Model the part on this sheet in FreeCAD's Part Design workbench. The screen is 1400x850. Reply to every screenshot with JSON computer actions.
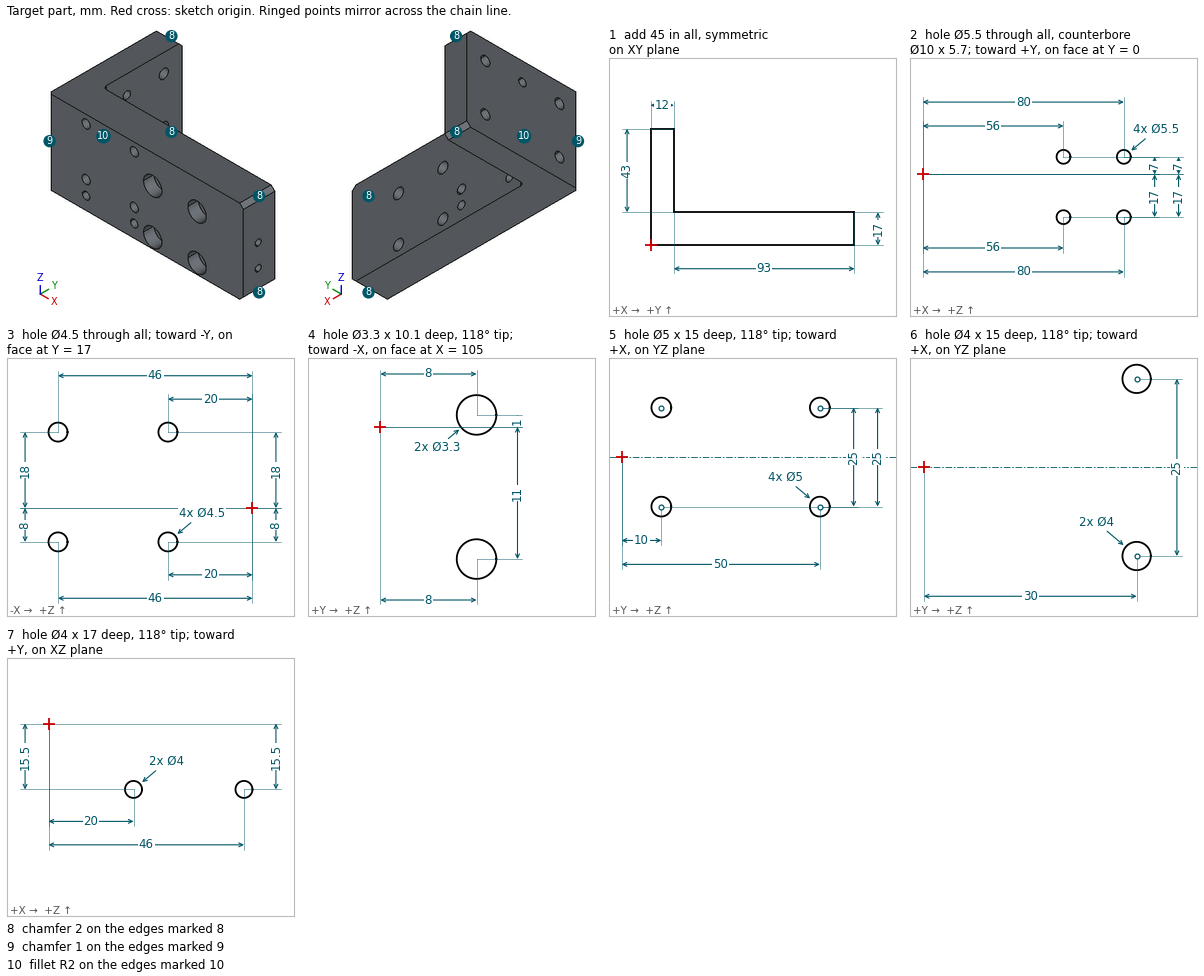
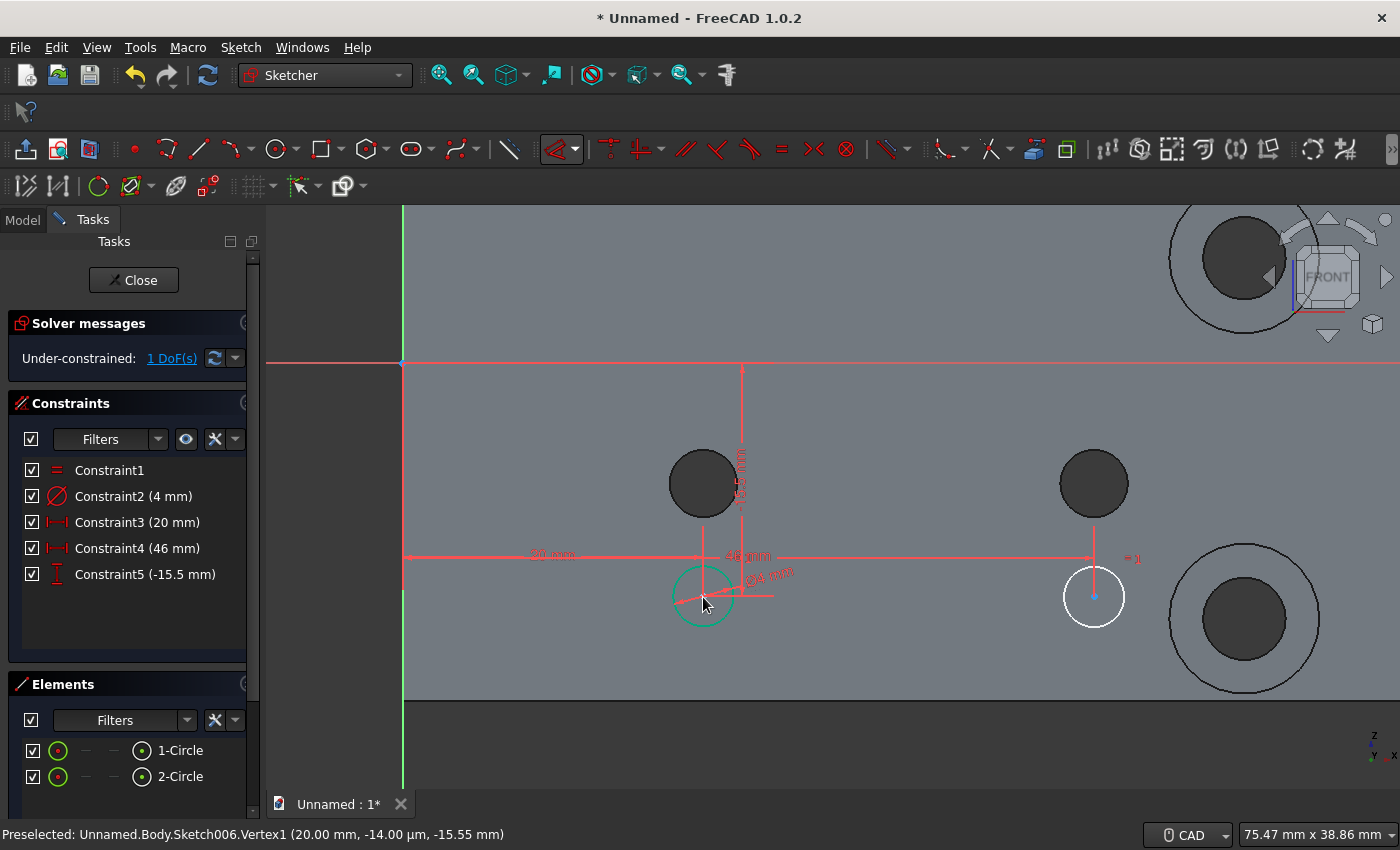
{"action": "left_click", "coordinate": [1094, 597]}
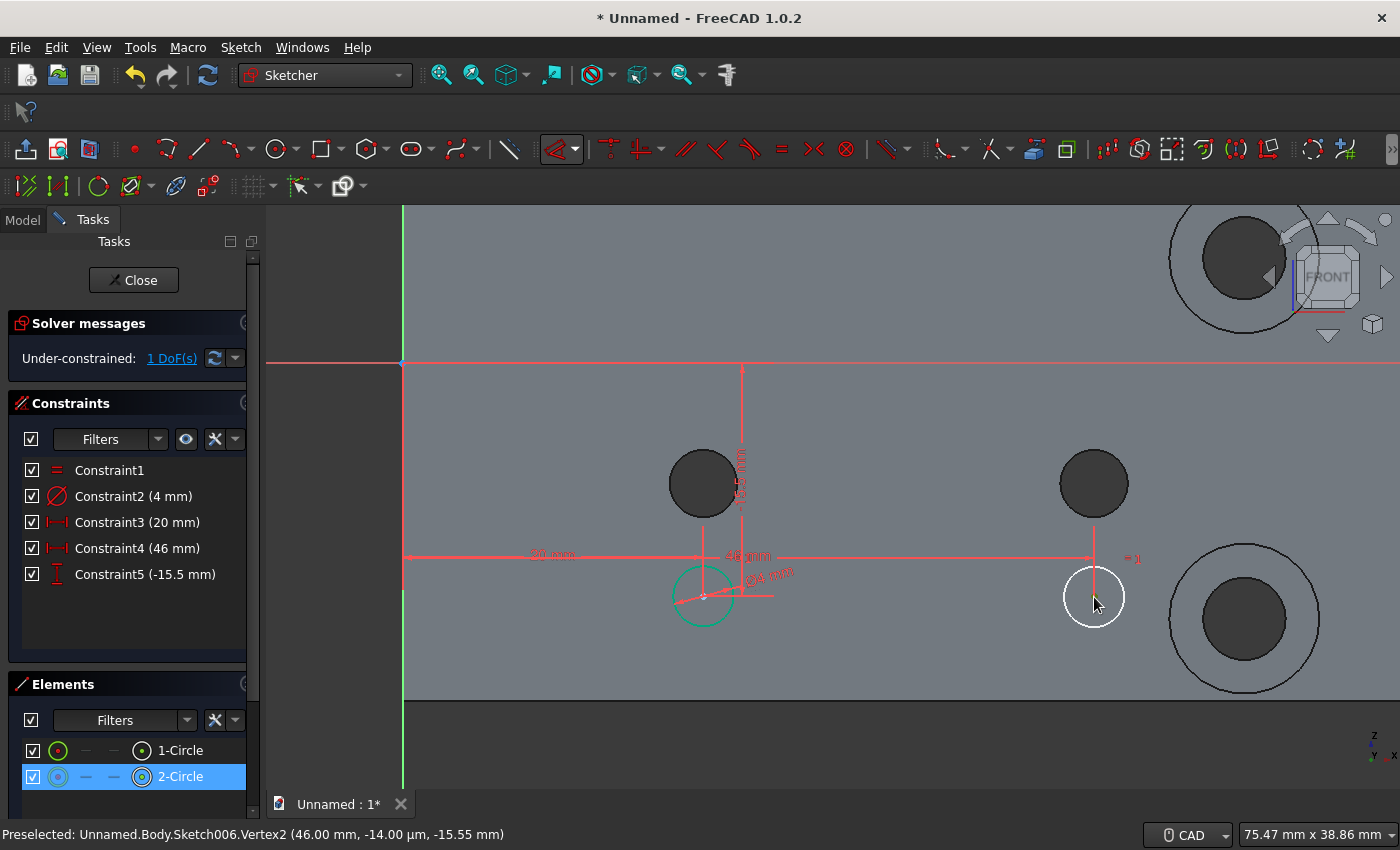
{"action": "key", "text": "i"}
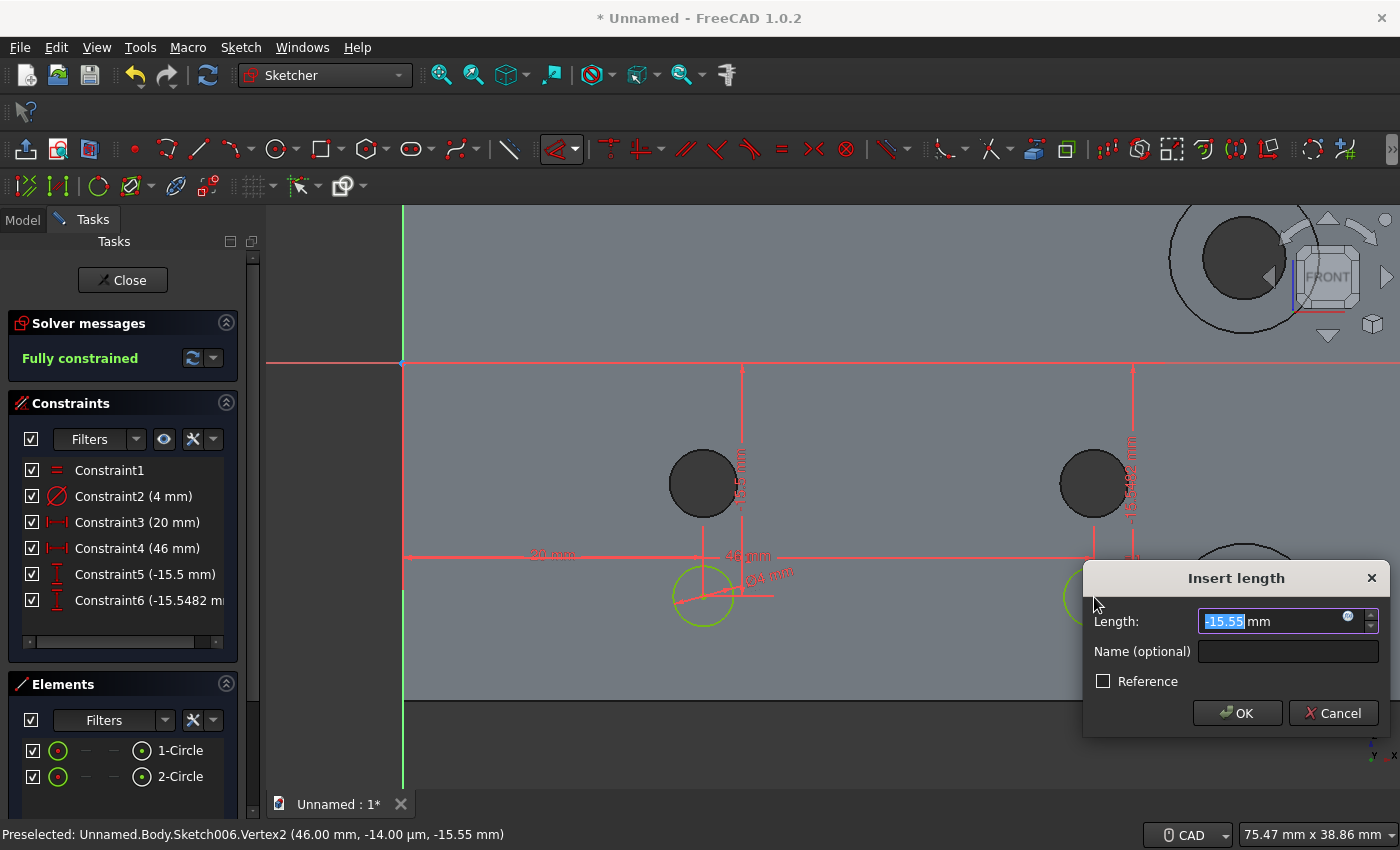
{"action": "type", "text": "-15.5"}
{"action": "key", "text": "Return"}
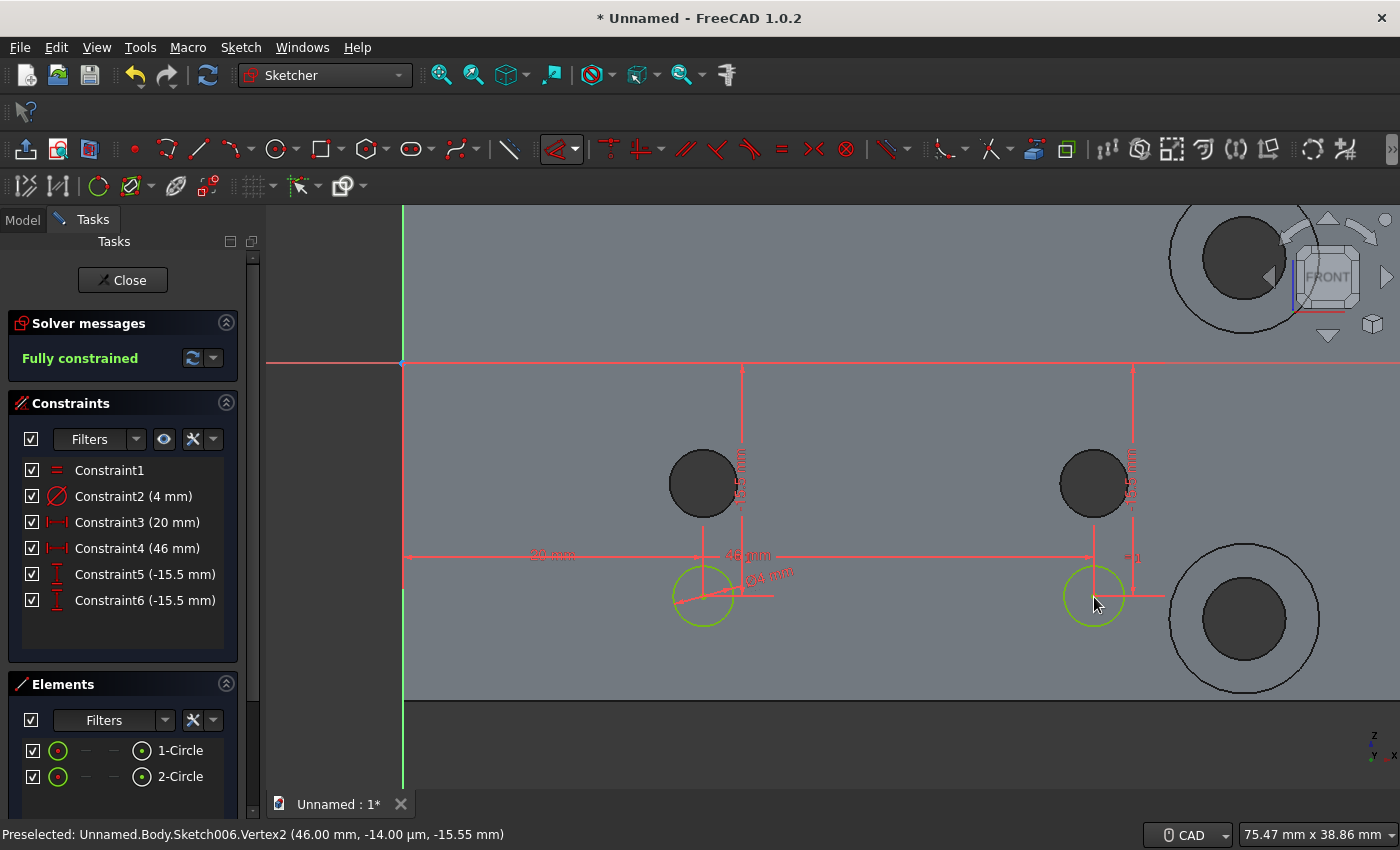
{"action": "left_click", "coordinate": [123, 280]}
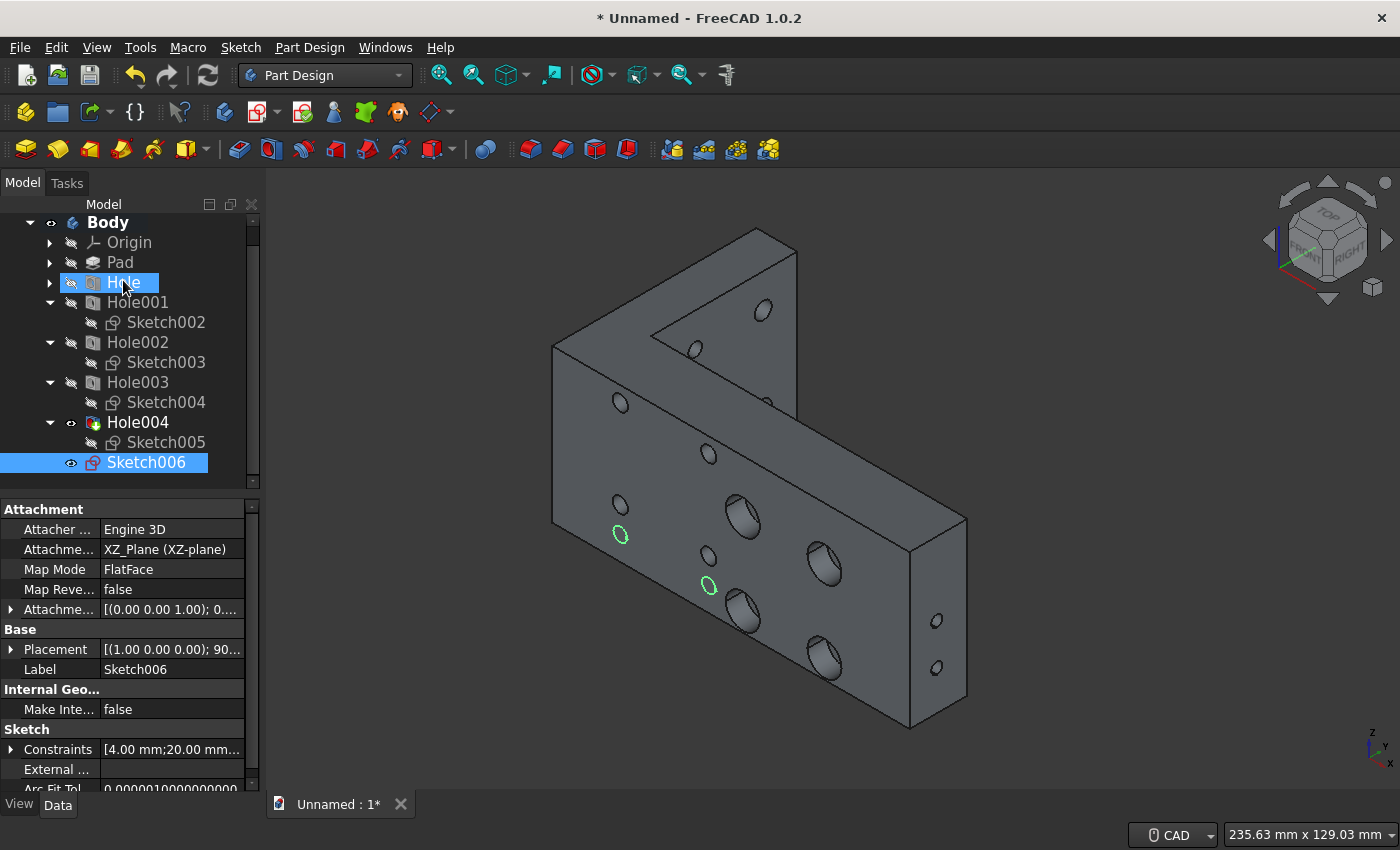
{"action": "left_click", "coordinate": [272, 150]}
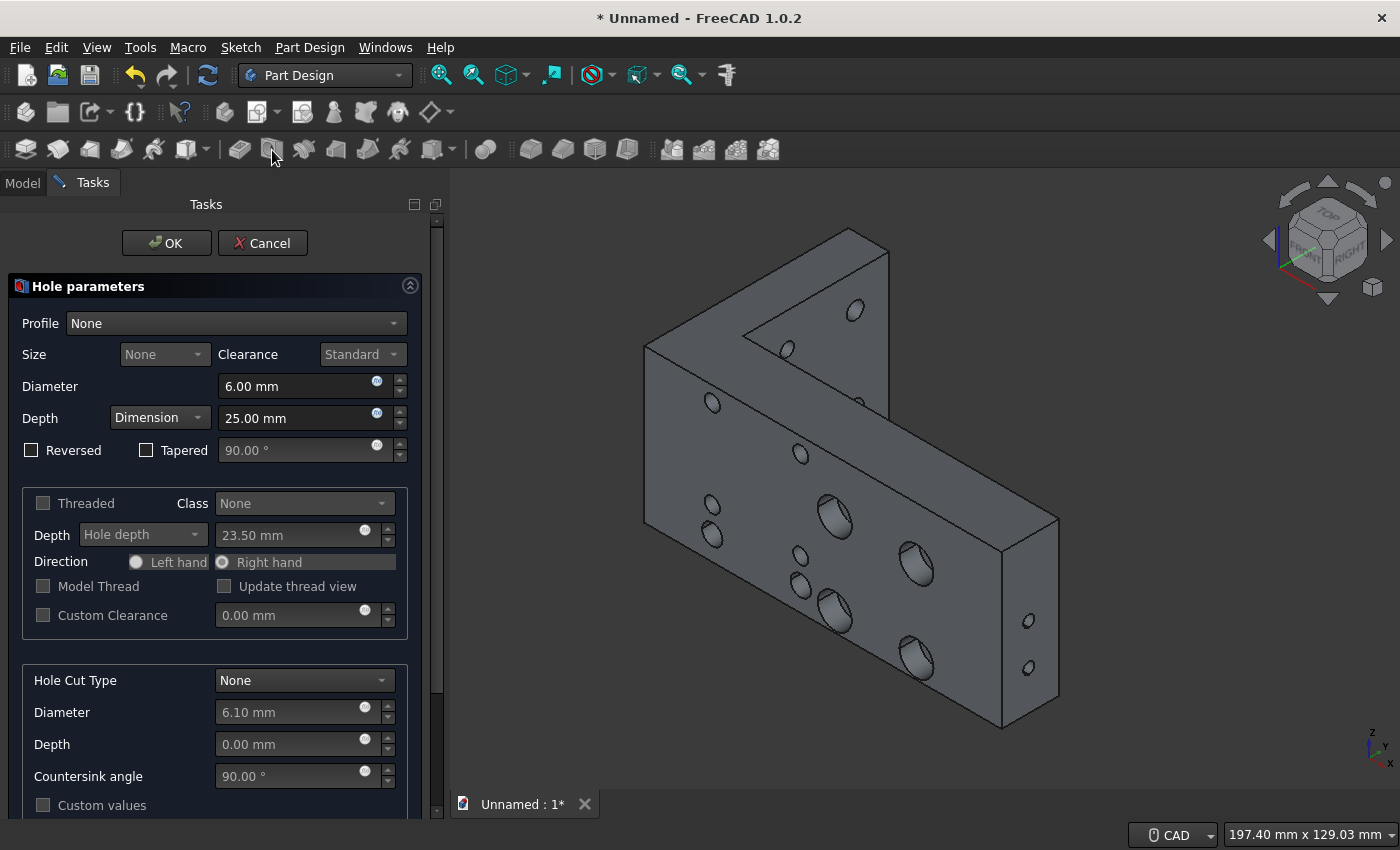
{"action": "triple_click", "coordinate": [305, 386]}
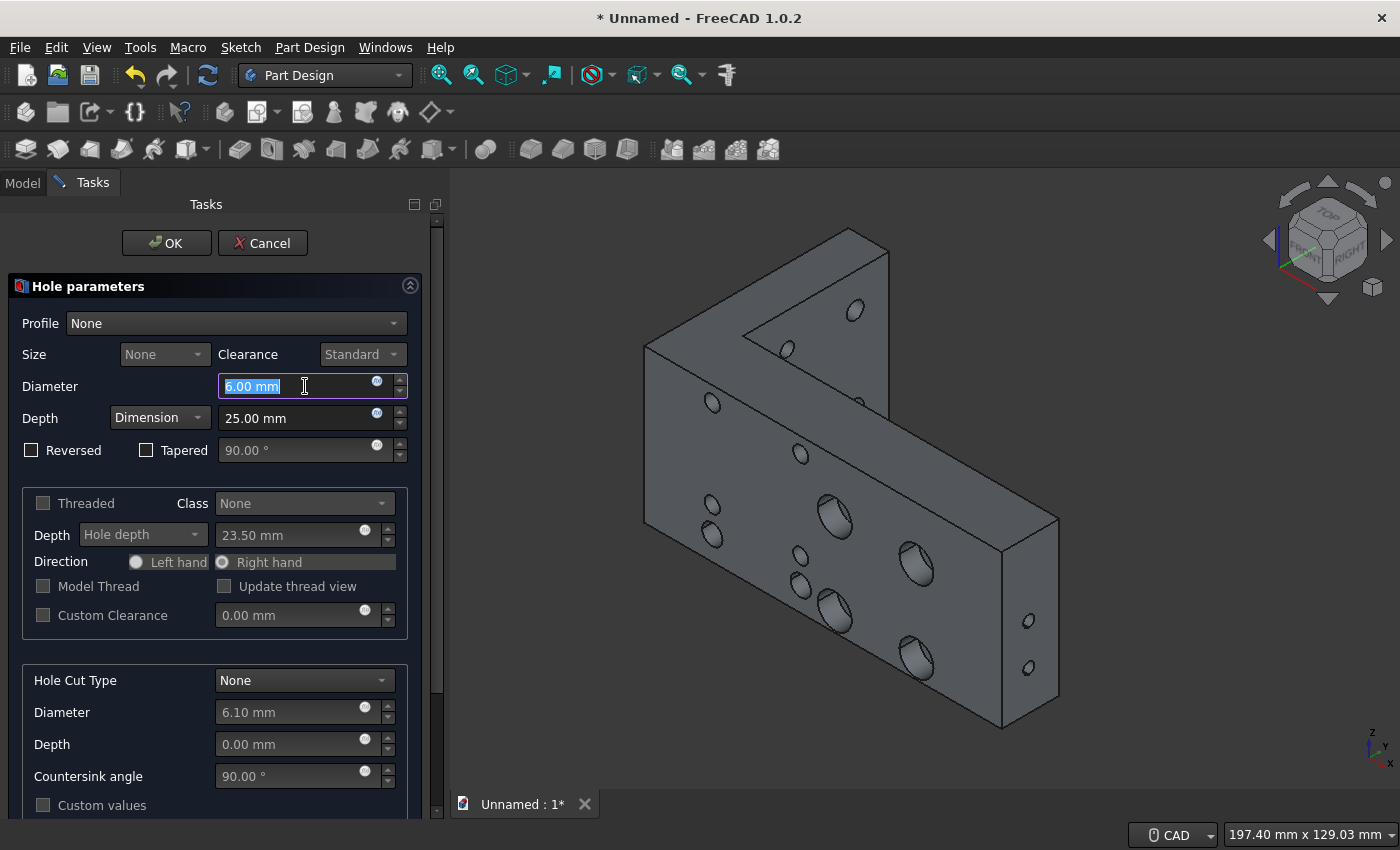
{"action": "type", "text": "4"}
{"action": "key", "text": "Tab"}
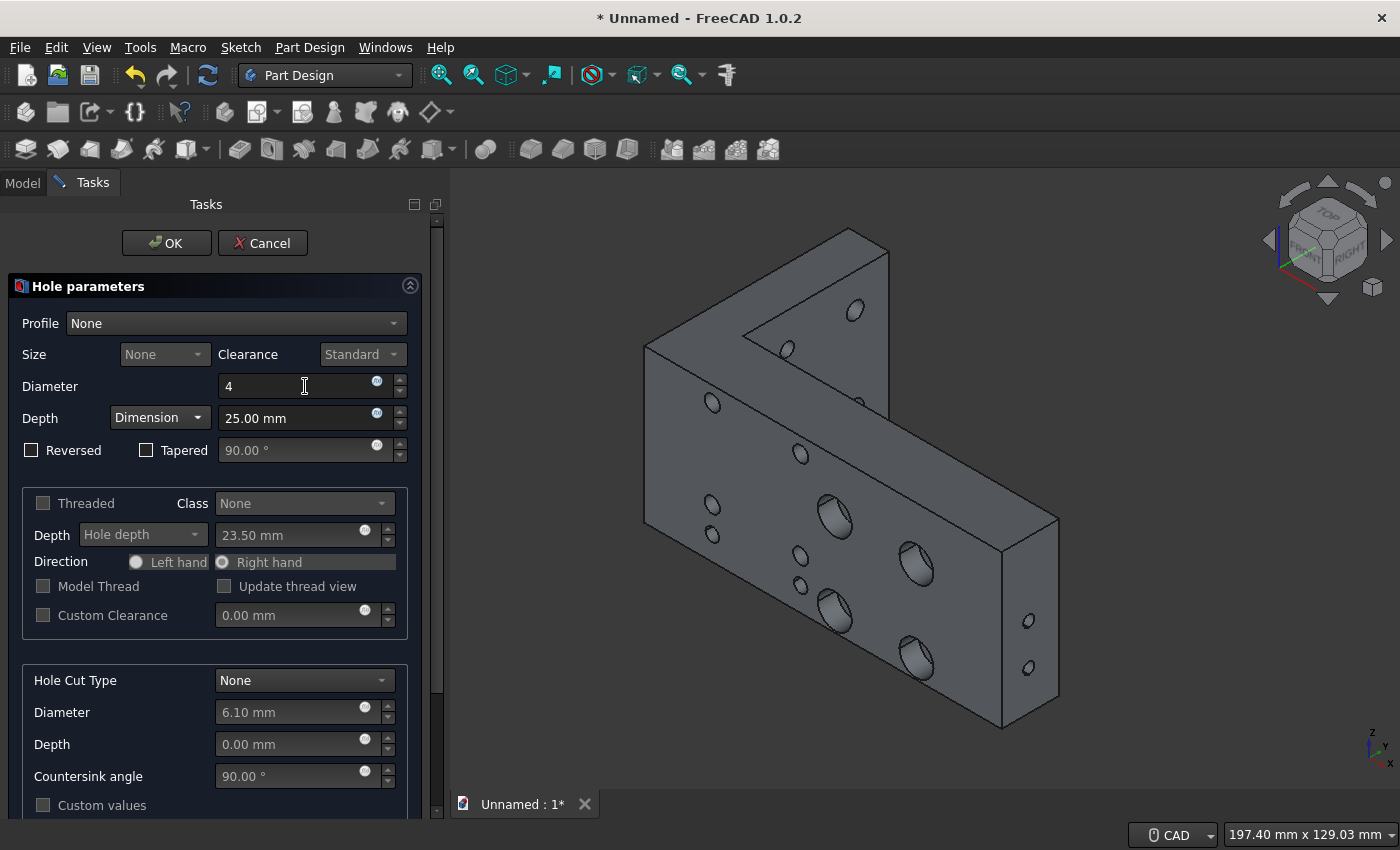
{"action": "triple_click", "coordinate": [305, 418]}